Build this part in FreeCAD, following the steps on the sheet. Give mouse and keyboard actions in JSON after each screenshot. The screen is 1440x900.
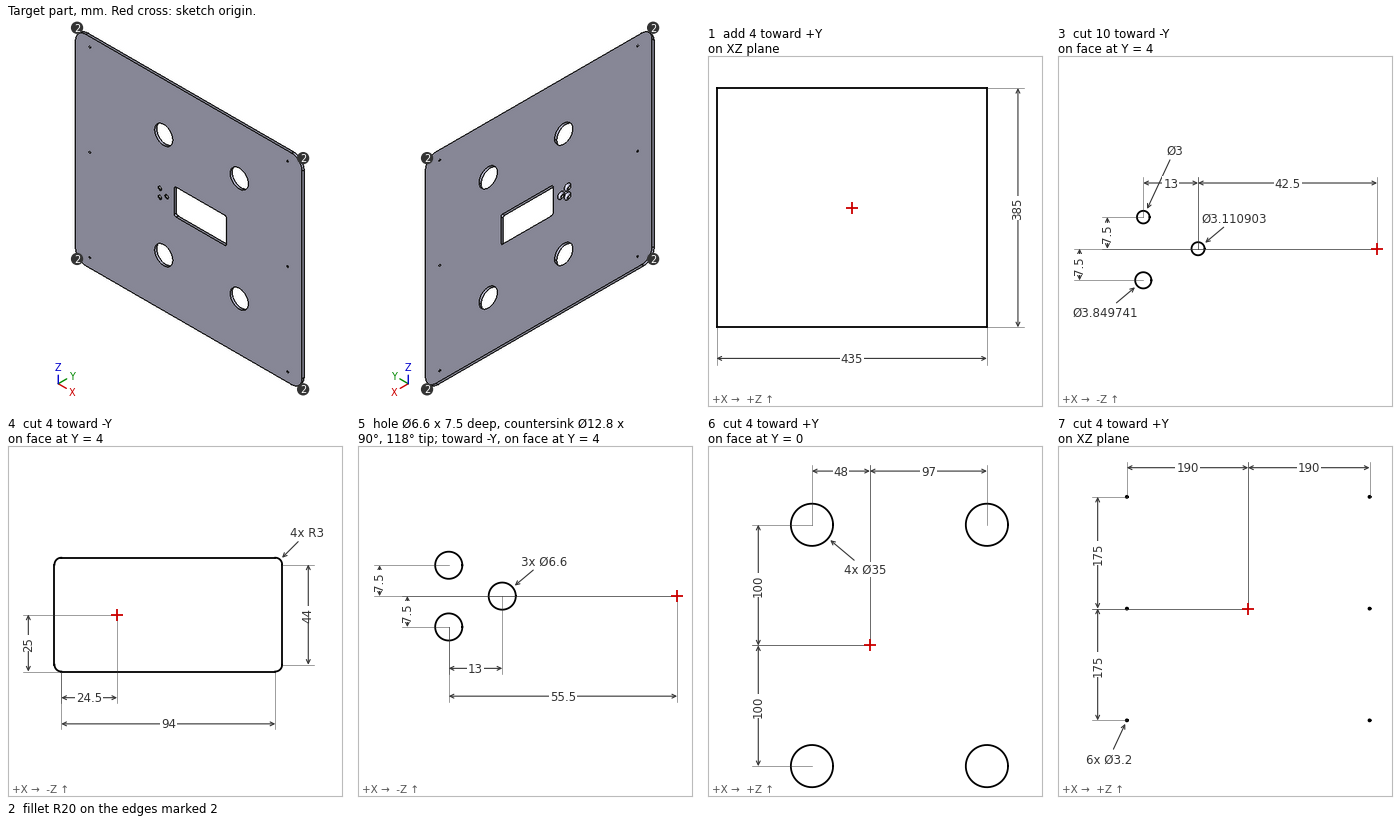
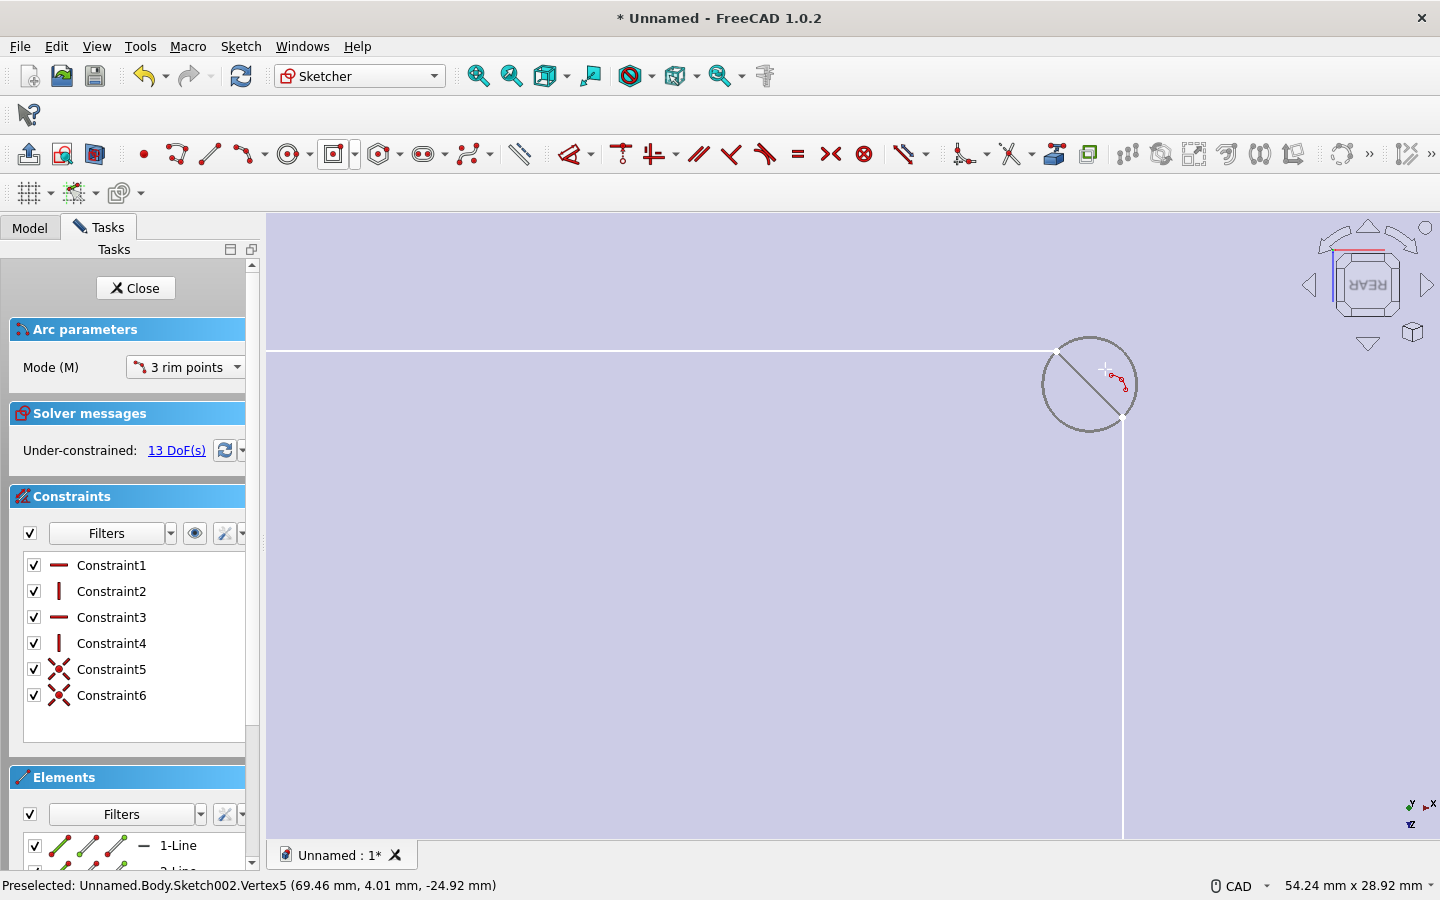
{"action": "left_click", "coordinate": [1103, 368]}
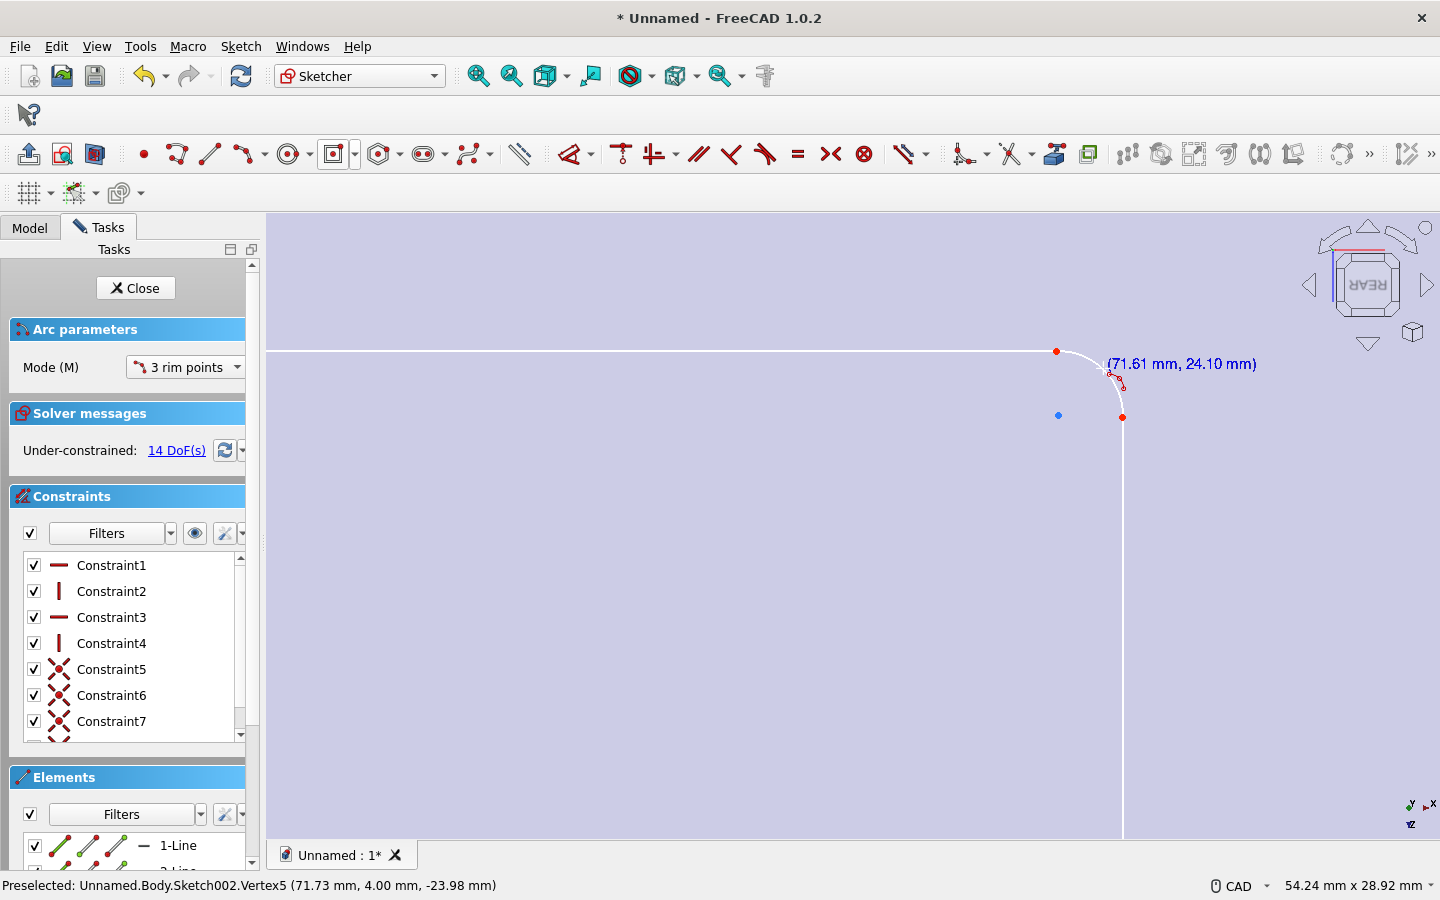
{"action": "scroll", "coordinate": [1105, 369], "scroll_direction": "down", "scroll_amount": 6}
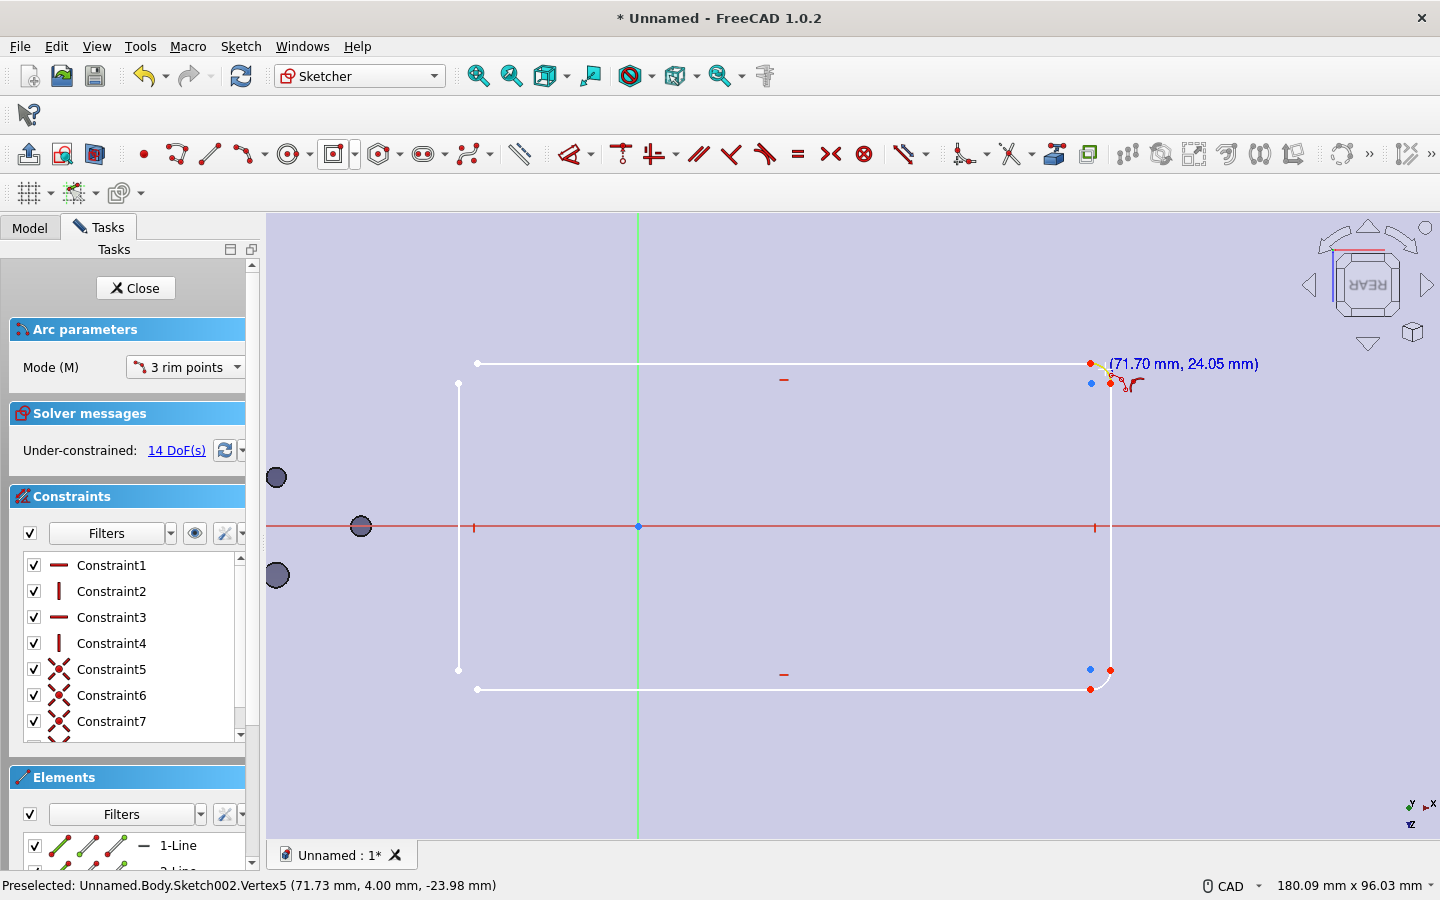
{"action": "left_click", "coordinate": [478, 364]}
{"action": "left_click", "coordinate": [459, 384]}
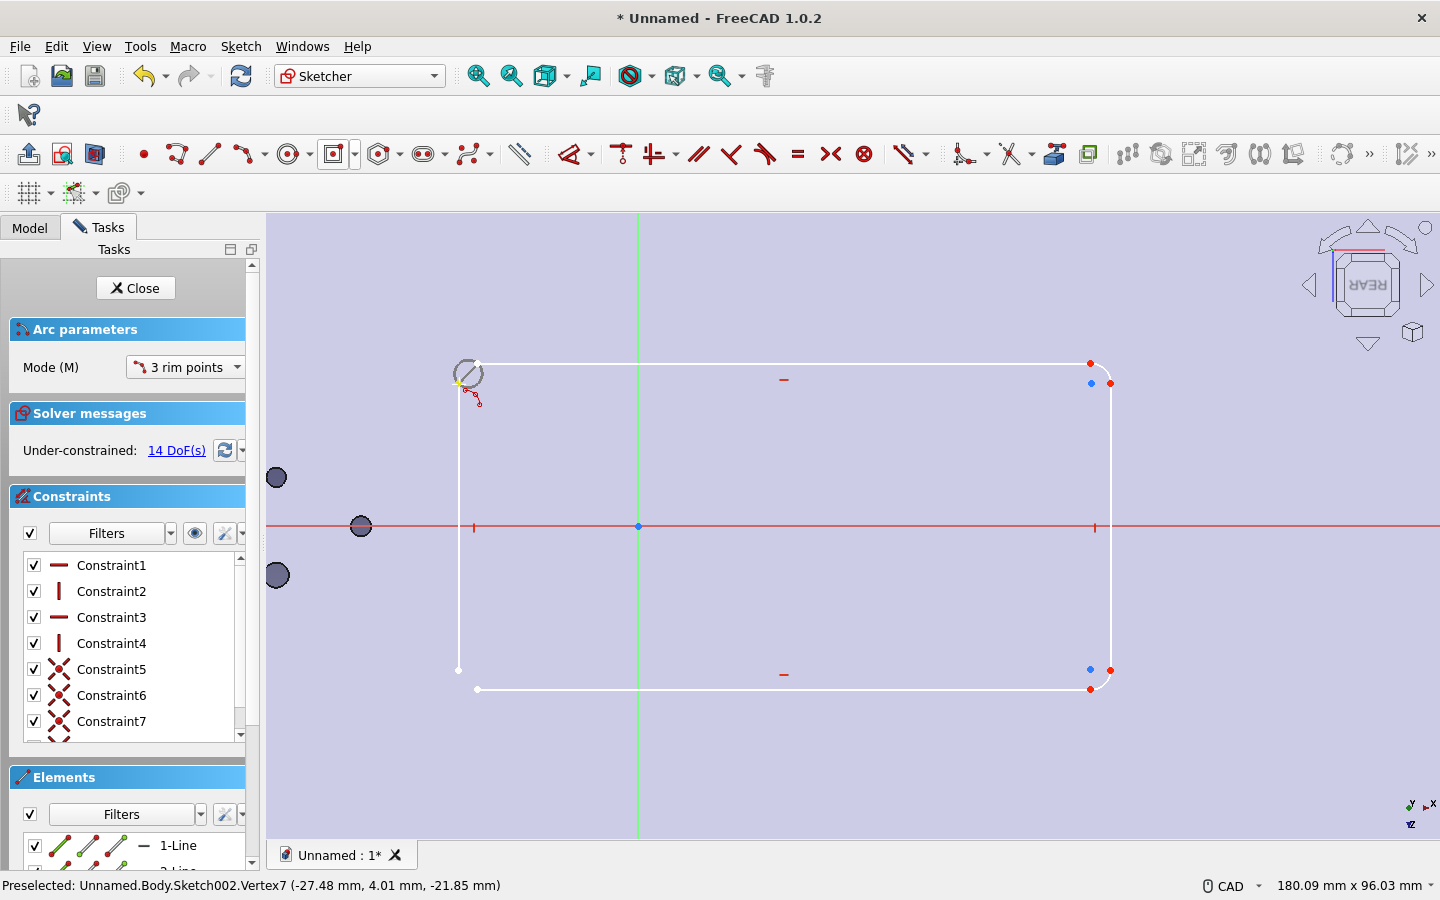
{"action": "scroll", "coordinate": [465, 369], "scroll_direction": "up", "scroll_amount": 6}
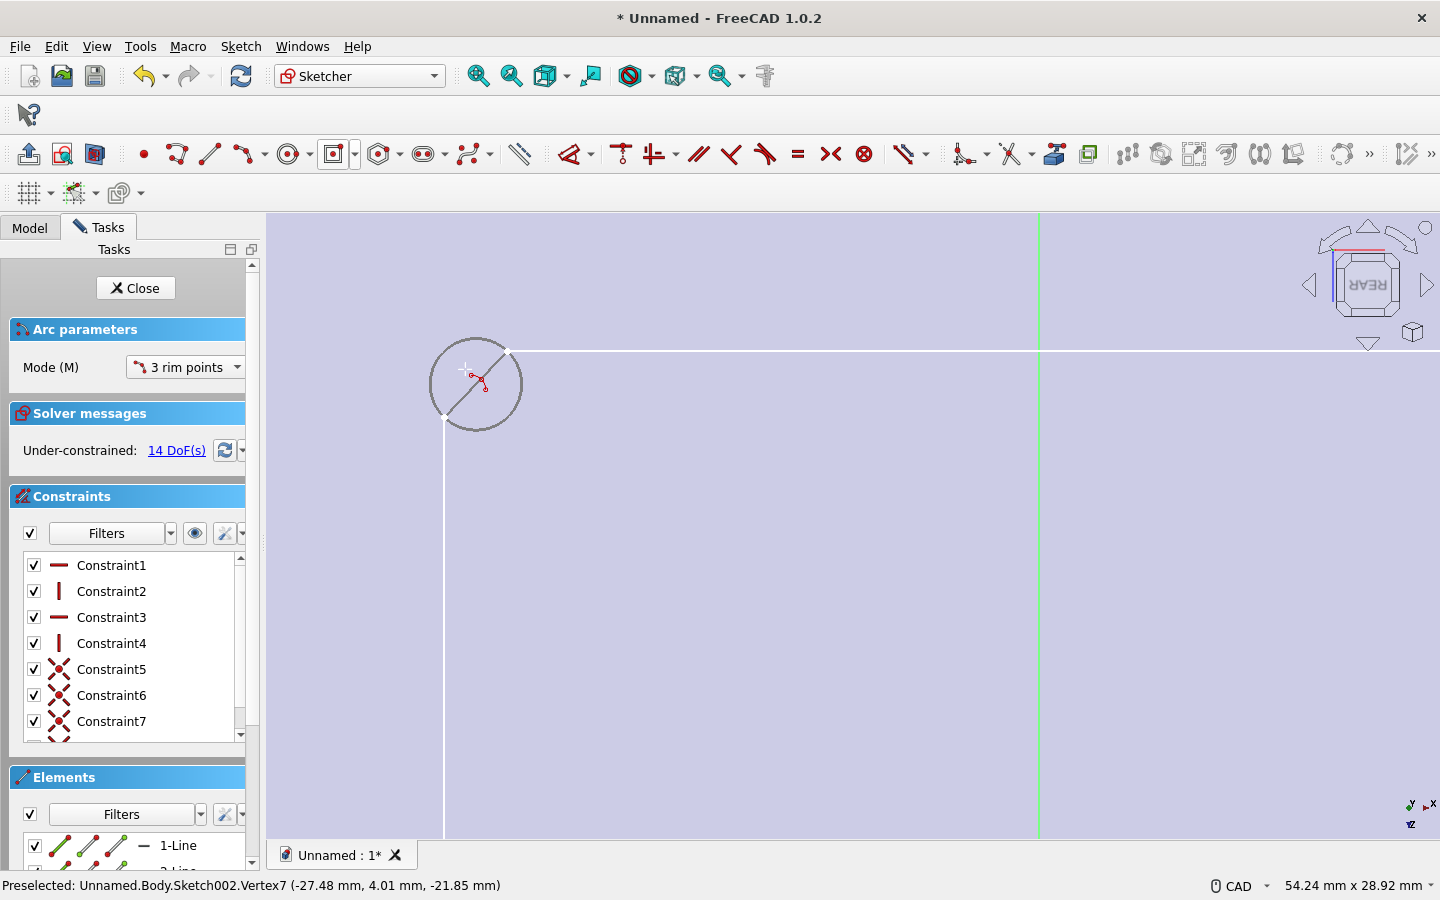
{"action": "left_click", "coordinate": [463, 368]}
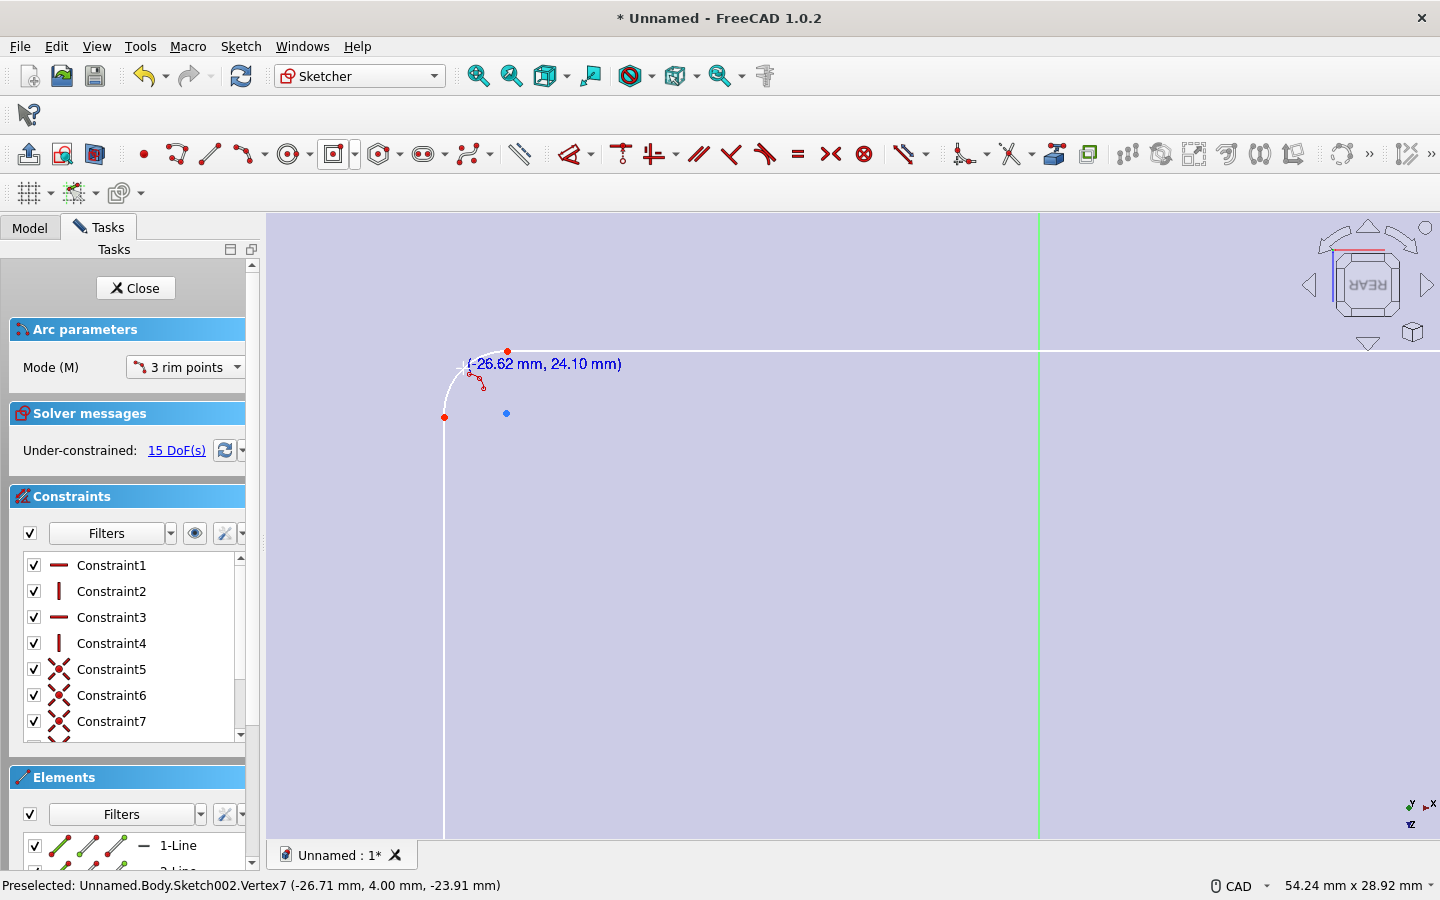
{"action": "scroll", "coordinate": [465, 369], "scroll_direction": "down", "scroll_amount": 6}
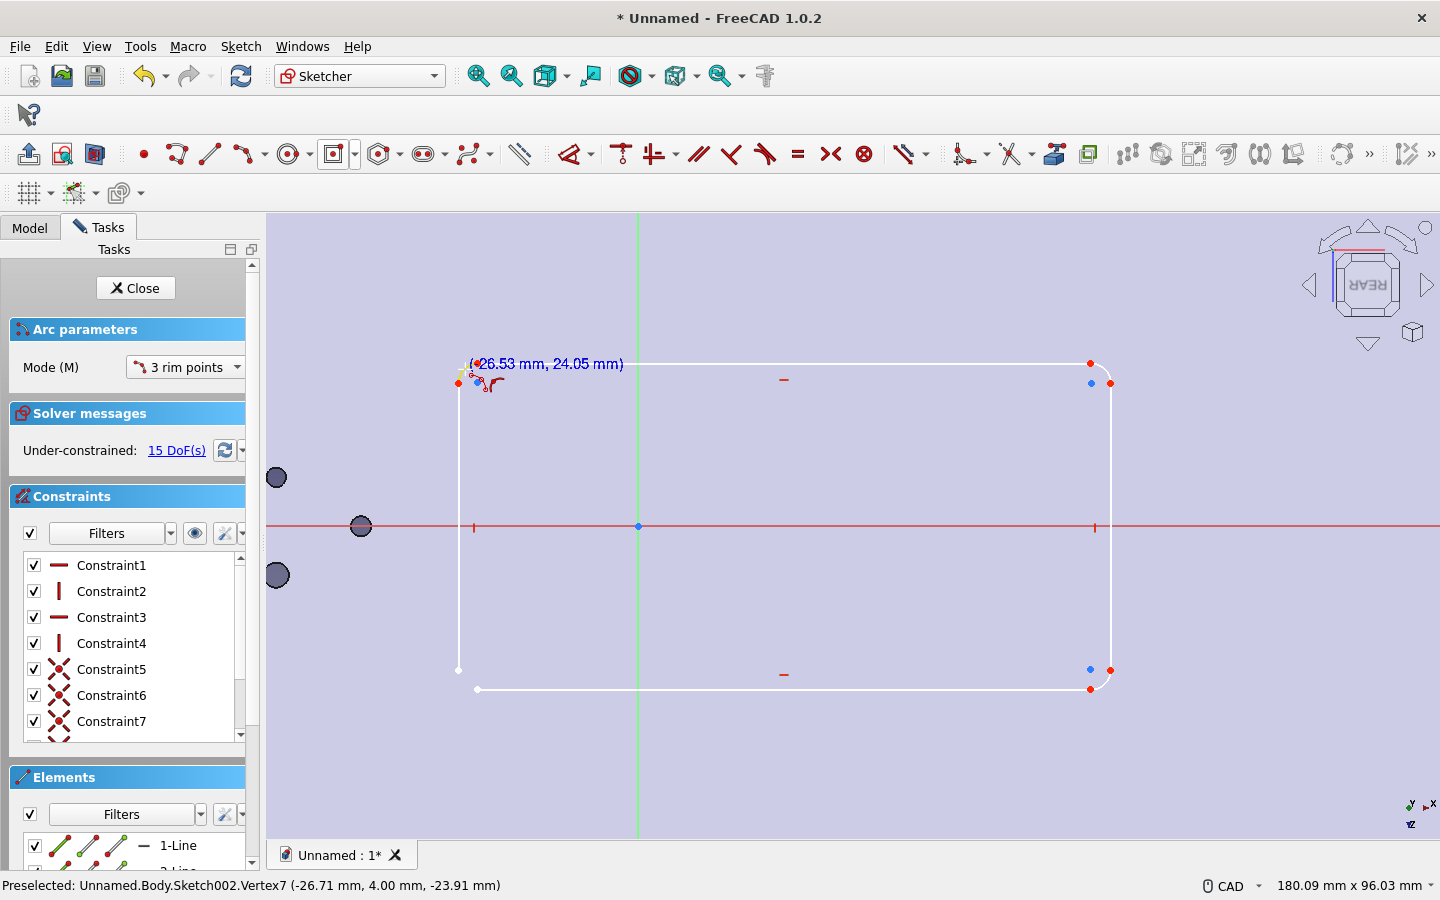
{"action": "left_click", "coordinate": [459, 671]}
{"action": "left_click", "coordinate": [478, 690]}